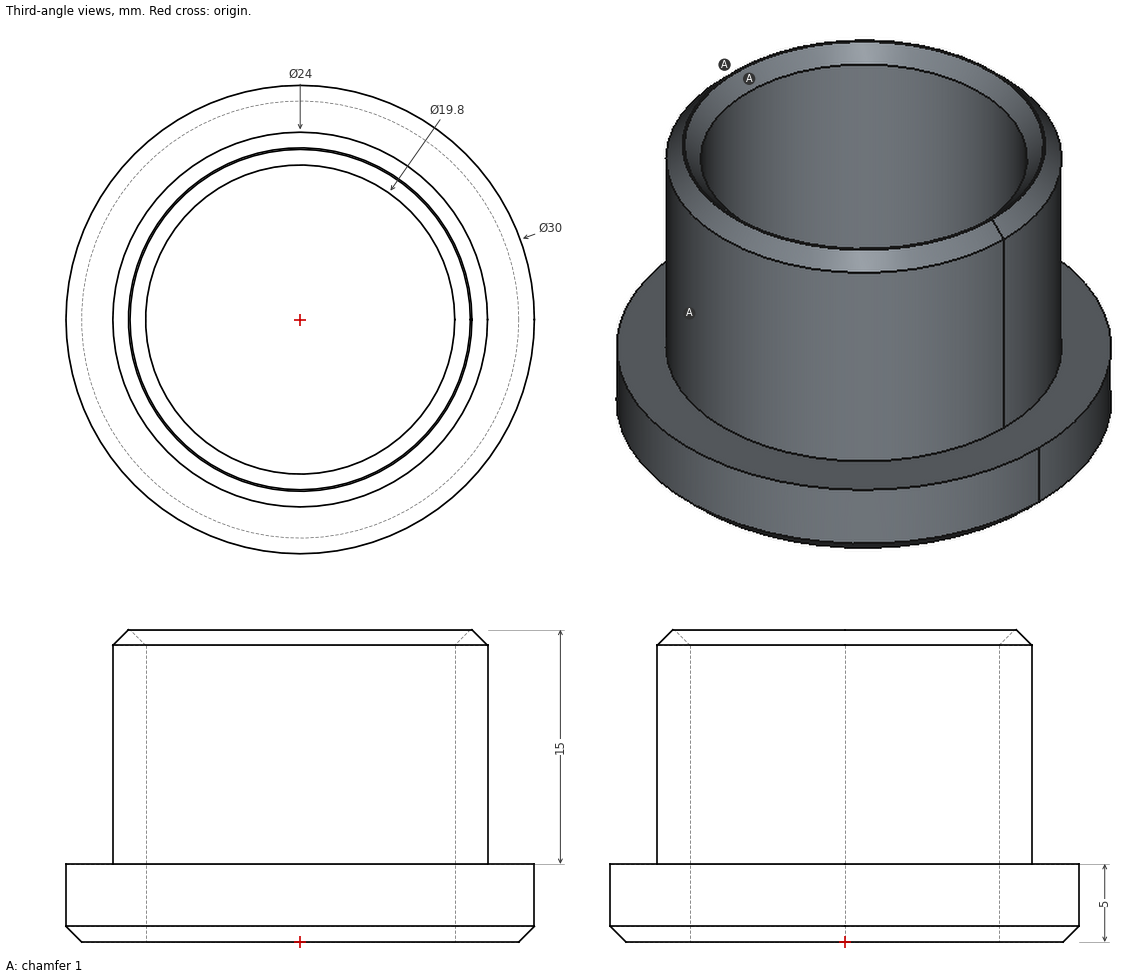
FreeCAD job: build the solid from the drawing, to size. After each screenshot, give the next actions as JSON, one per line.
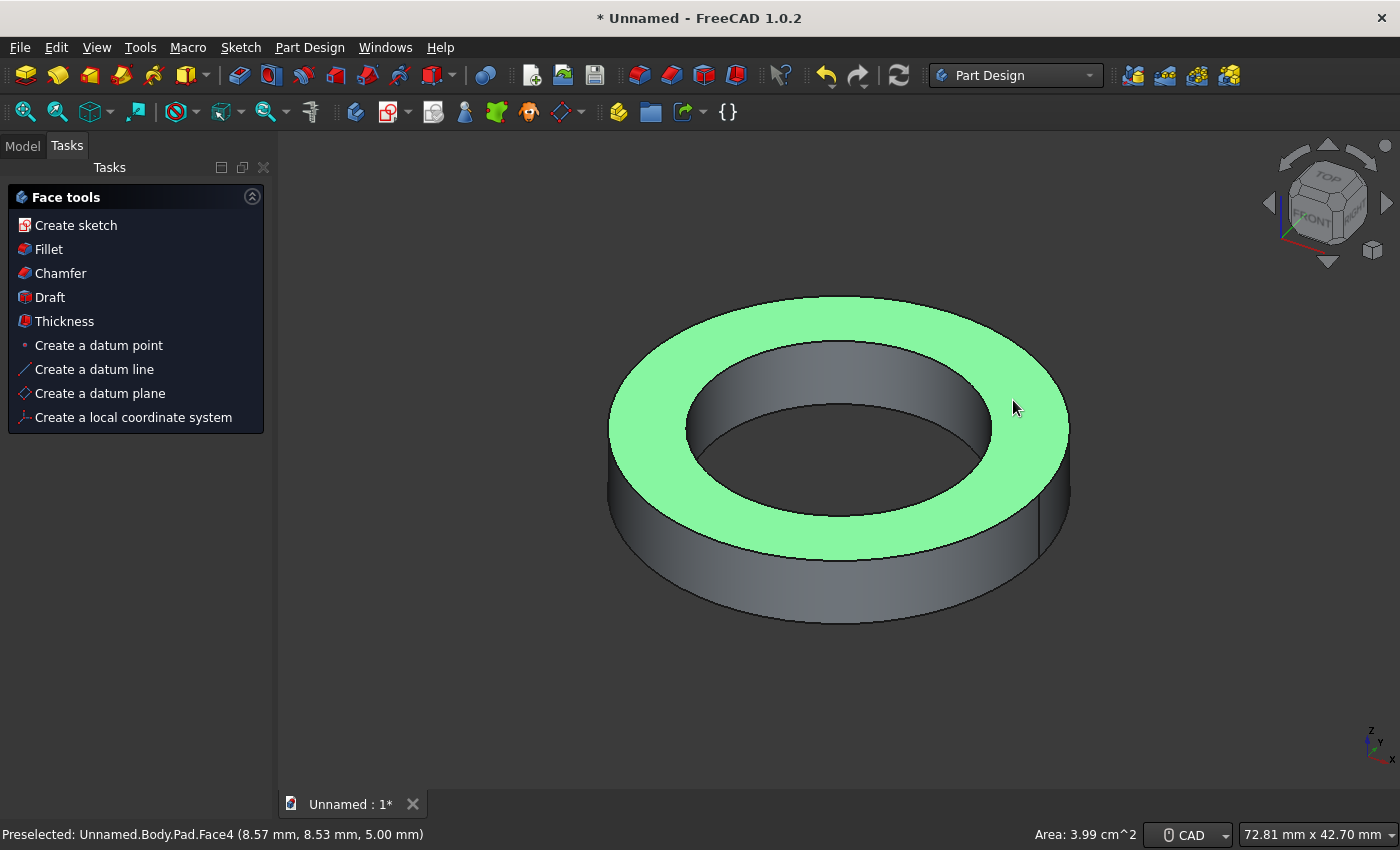
{"action": "left_click", "coordinate": [388, 112]}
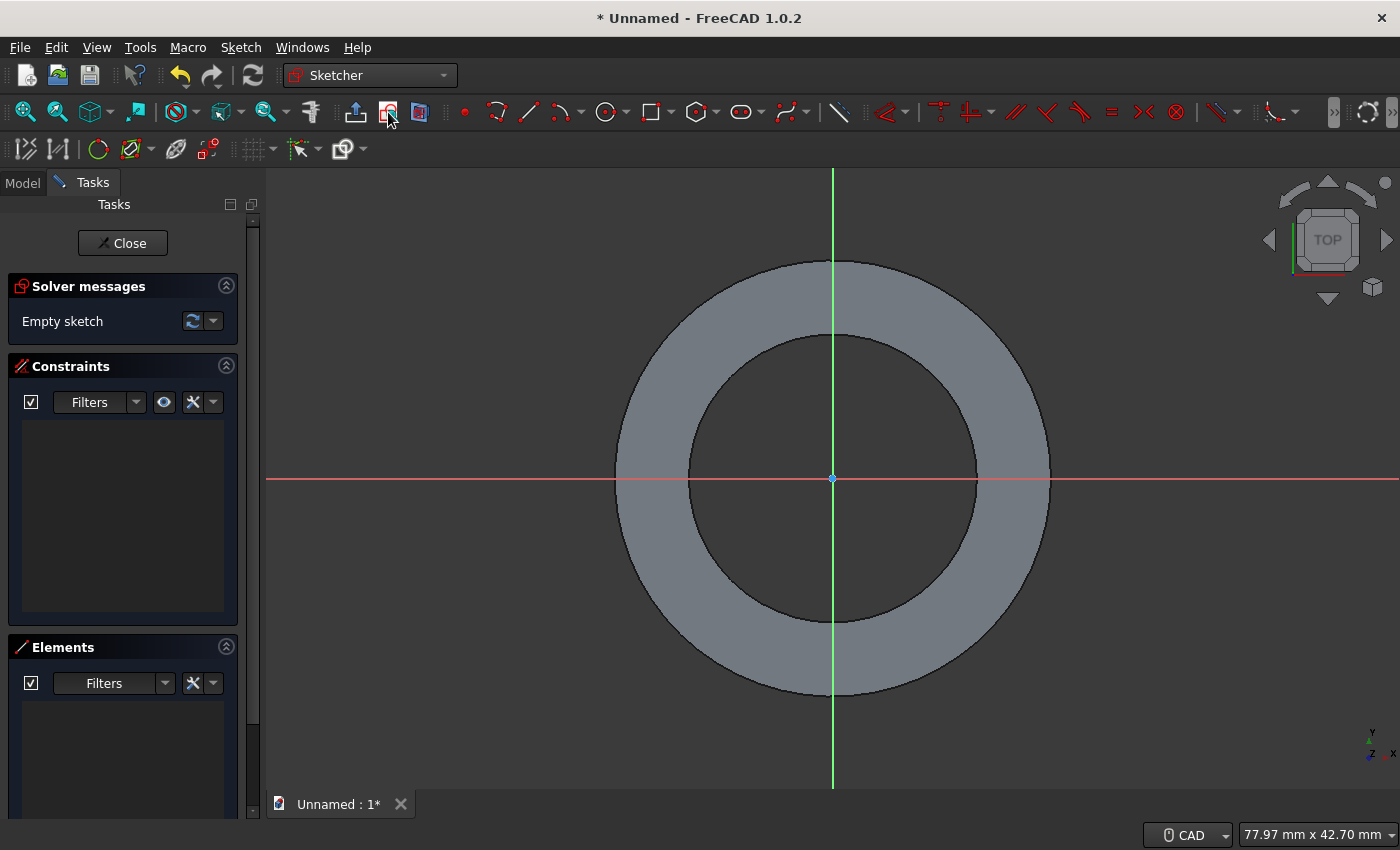
{"action": "left_click", "coordinate": [606, 112]}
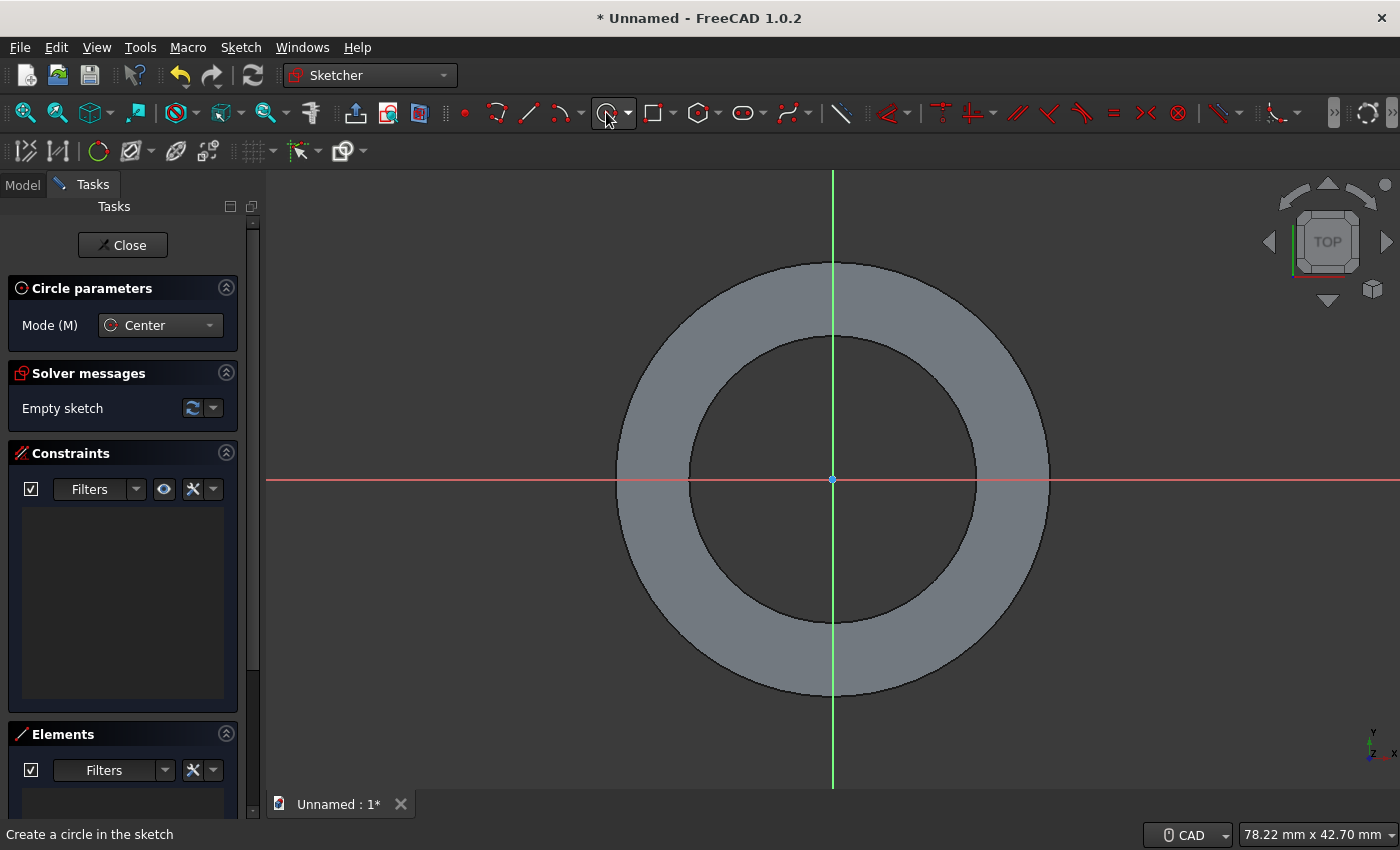
{"action": "left_click", "coordinate": [833, 480]}
{"action": "mouse_move", "coordinate": [956, 356]}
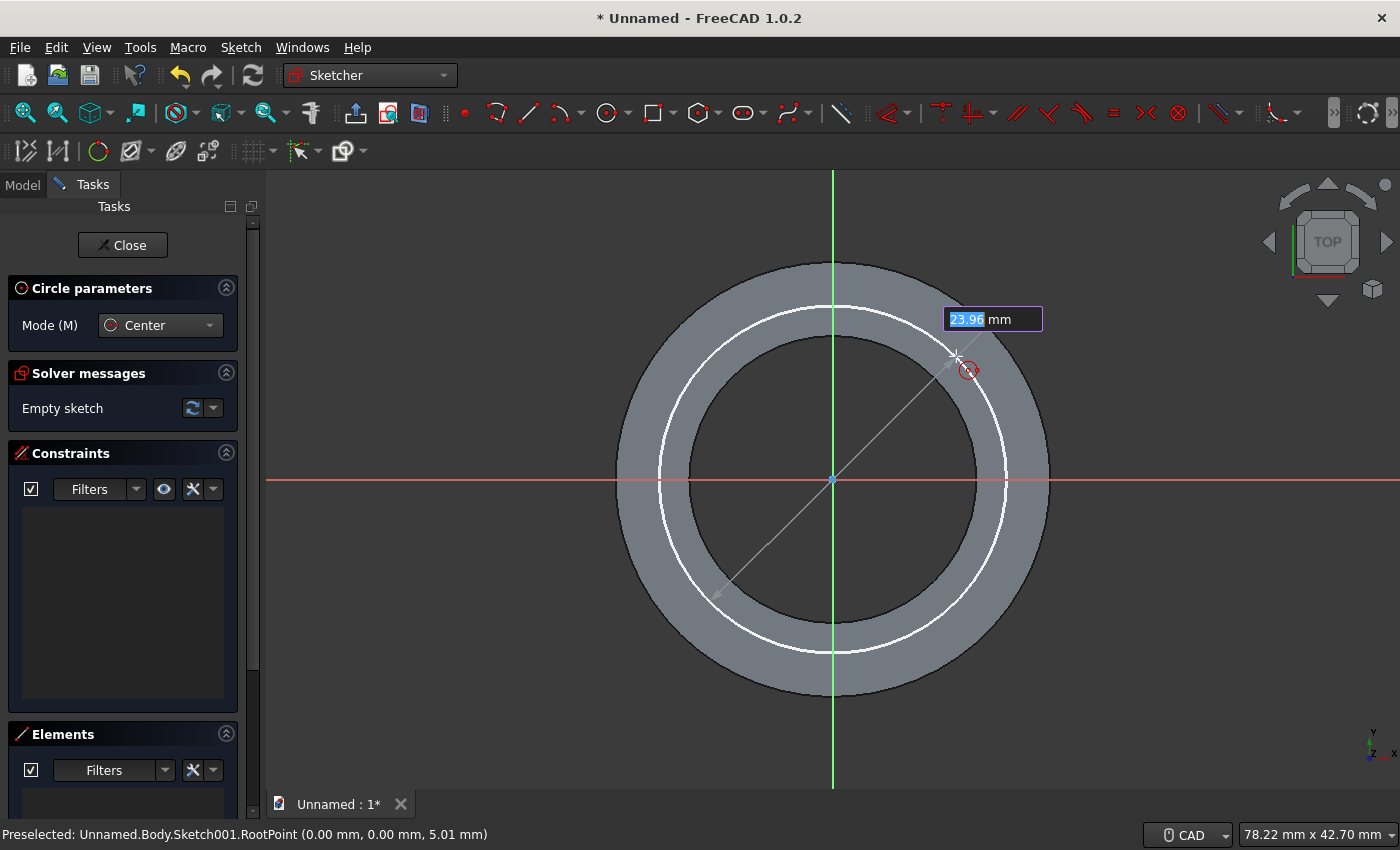
{"action": "type", "text": "24"}
{"action": "key", "text": "Return"}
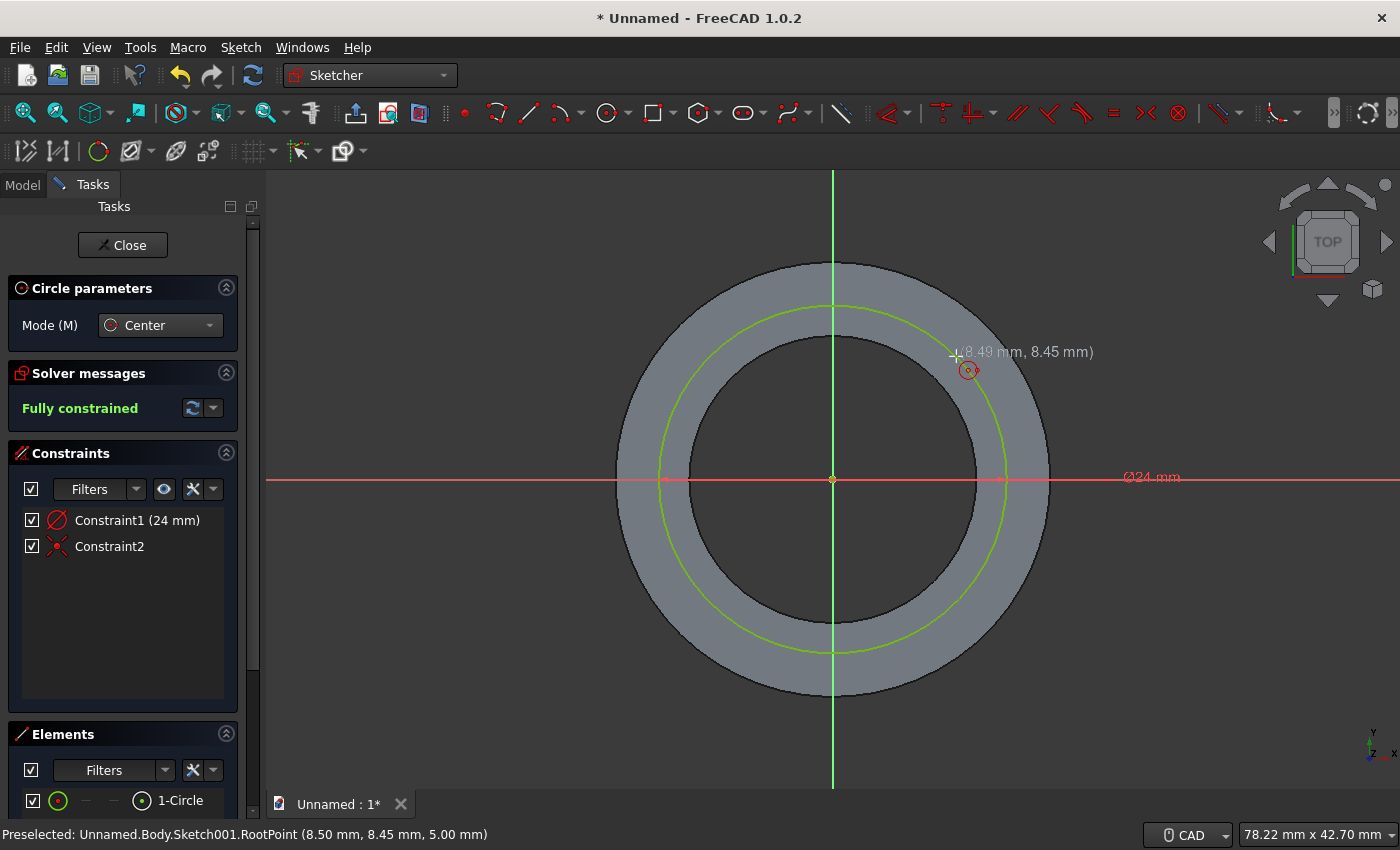
{"action": "left_click", "coordinate": [833, 480]}
{"action": "mouse_move", "coordinate": [934, 378]}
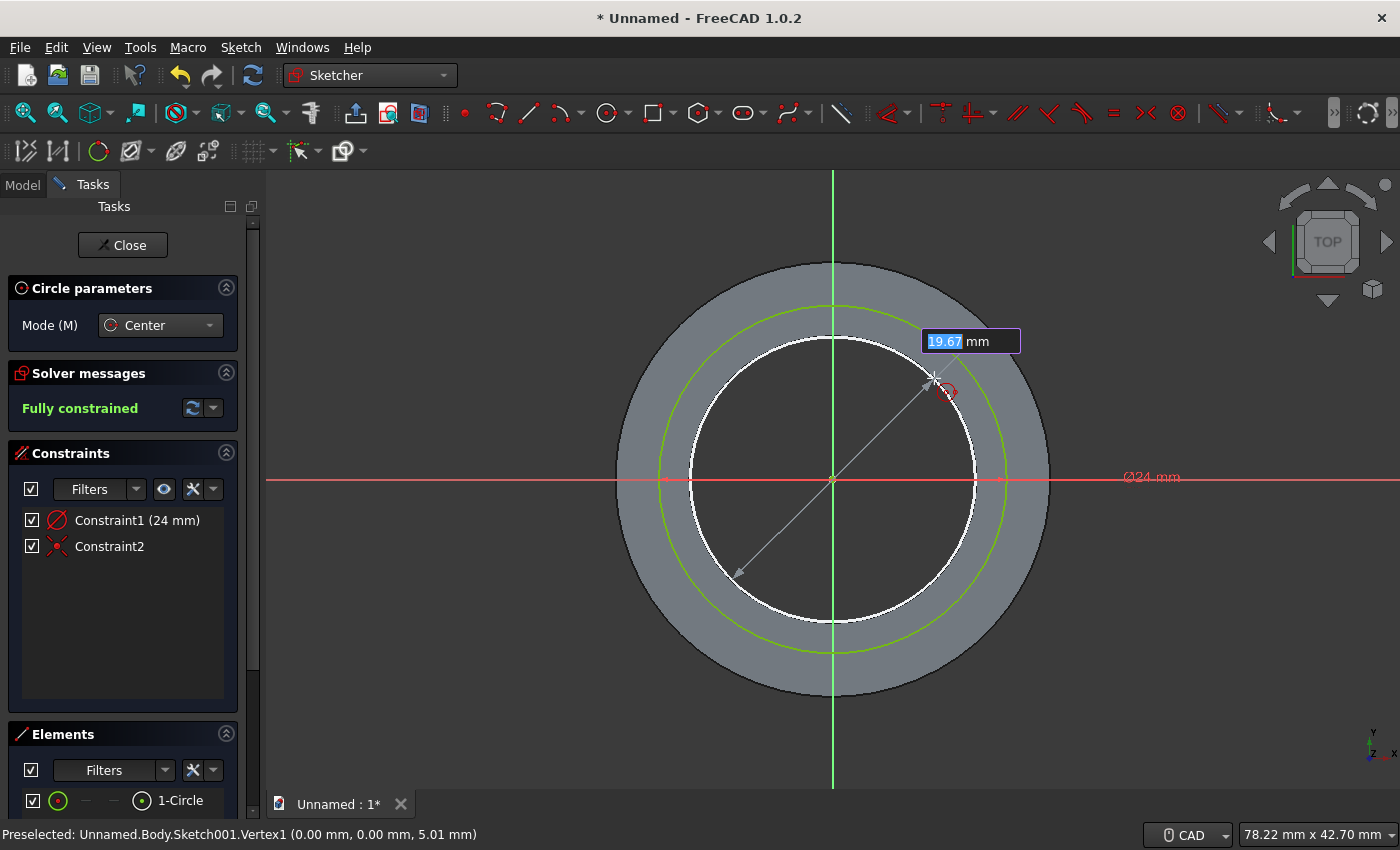
{"action": "type", "text": "19.8"}
{"action": "key", "text": "Return"}
{"action": "key", "text": "Escape"}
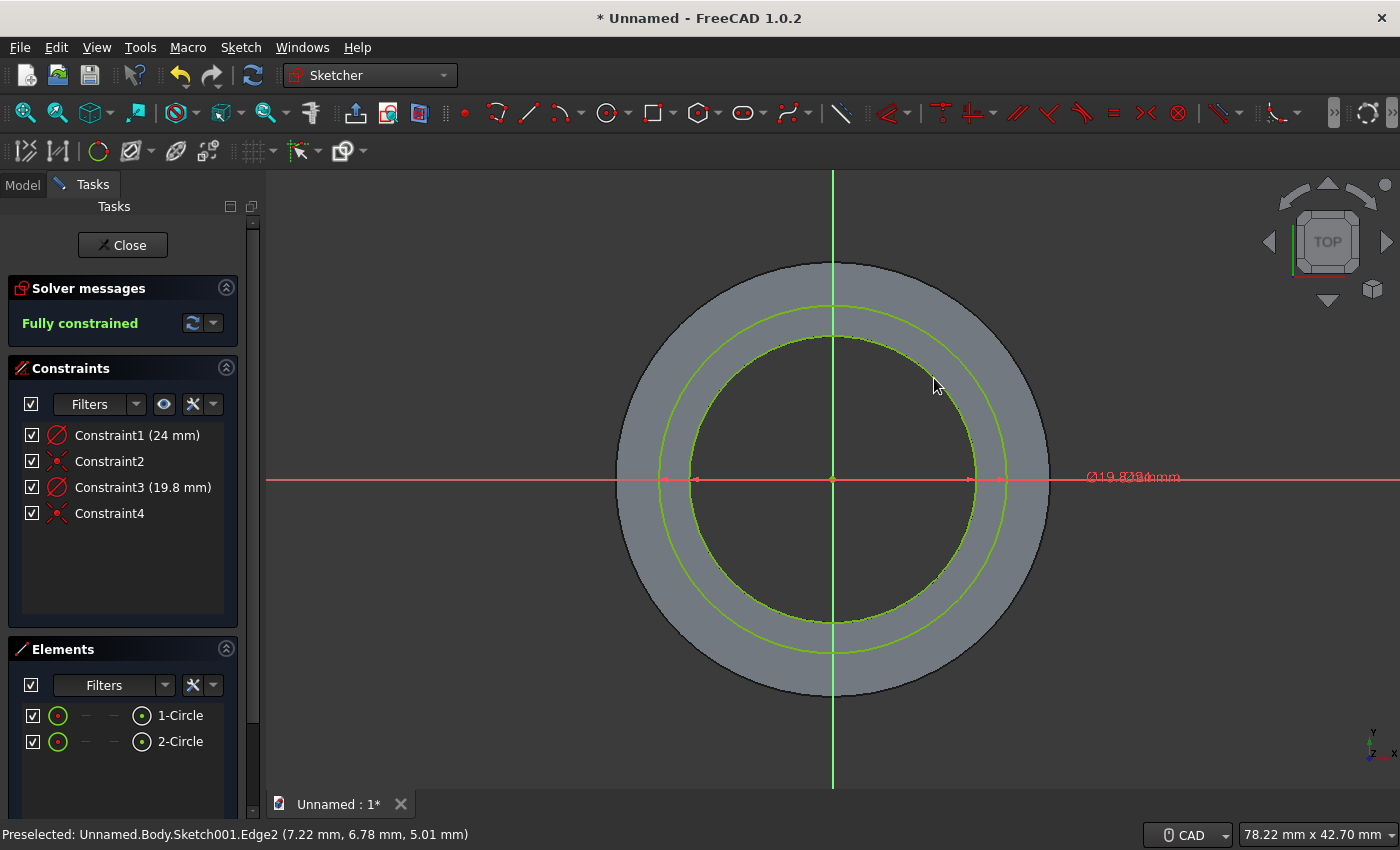
{"action": "left_click", "coordinate": [123, 245]}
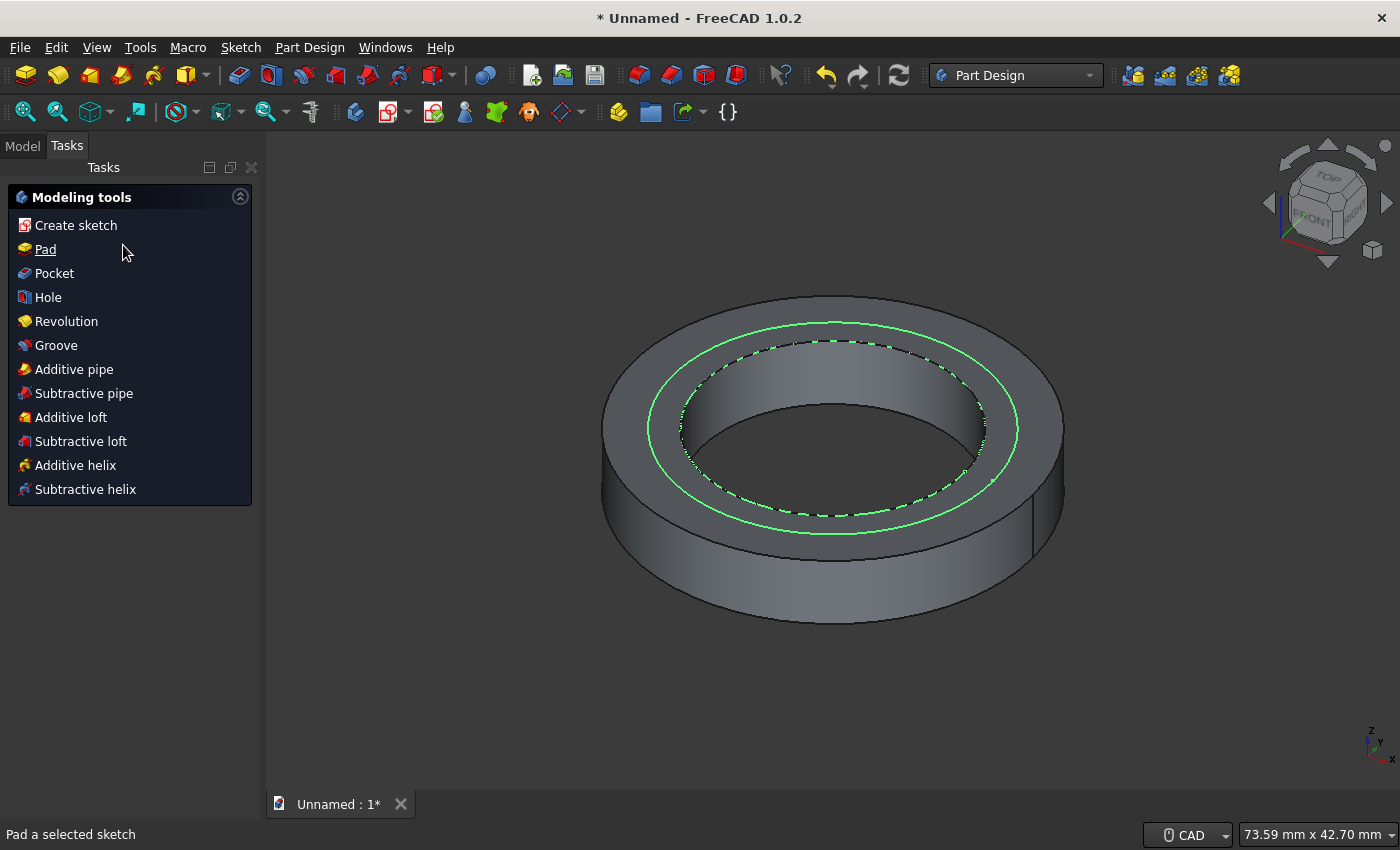
{"action": "left_click", "coordinate": [26, 76]}